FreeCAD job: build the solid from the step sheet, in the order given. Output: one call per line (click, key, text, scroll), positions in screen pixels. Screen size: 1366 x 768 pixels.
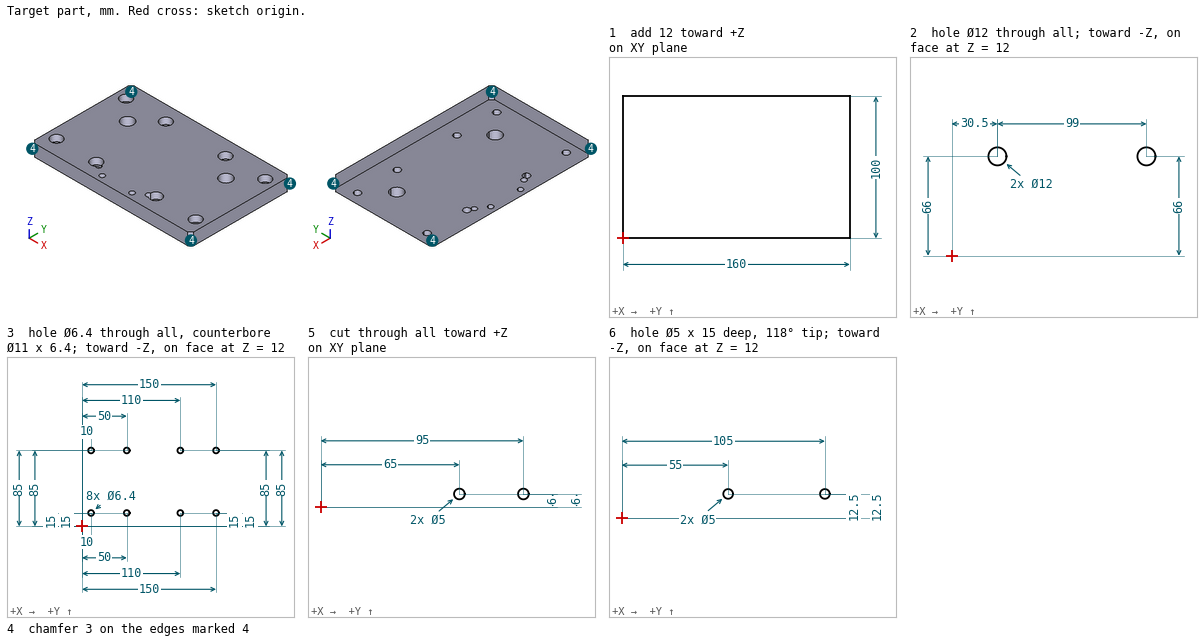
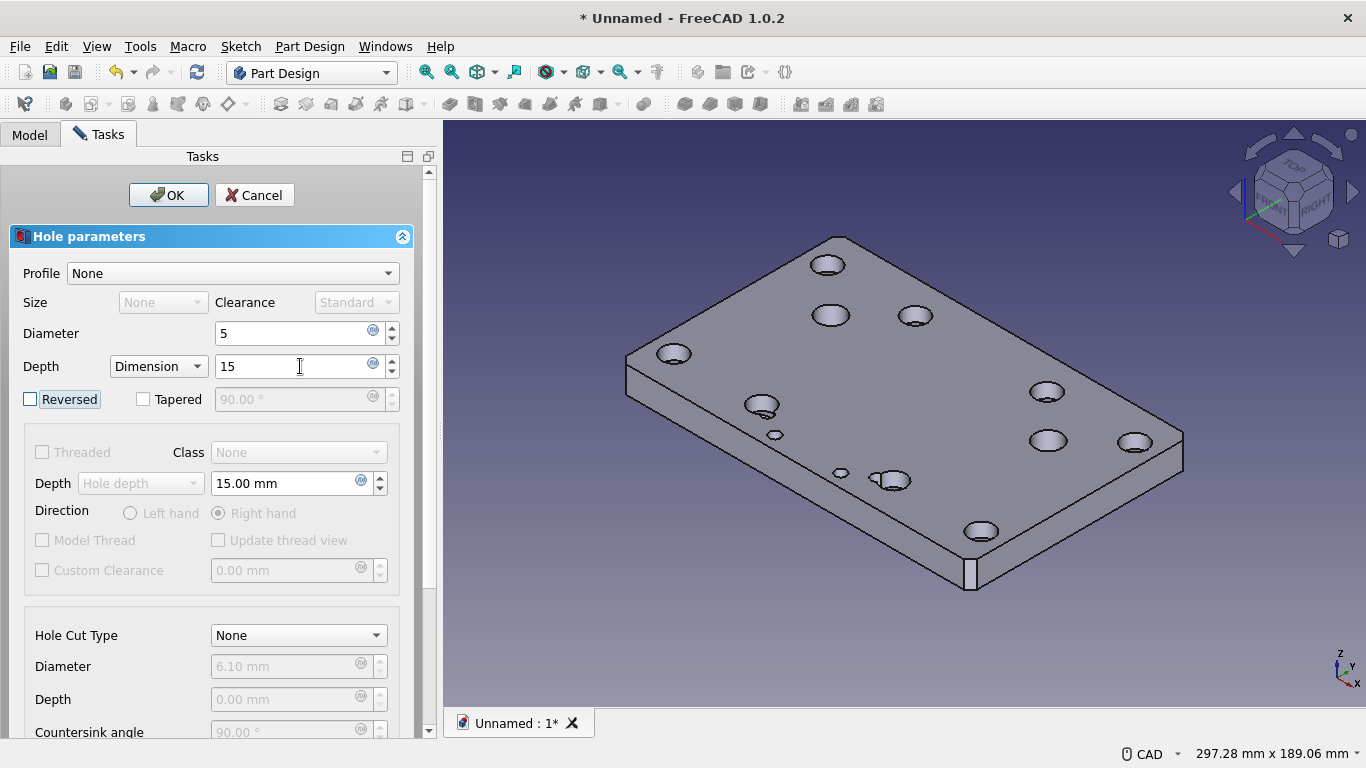
click(169, 195)